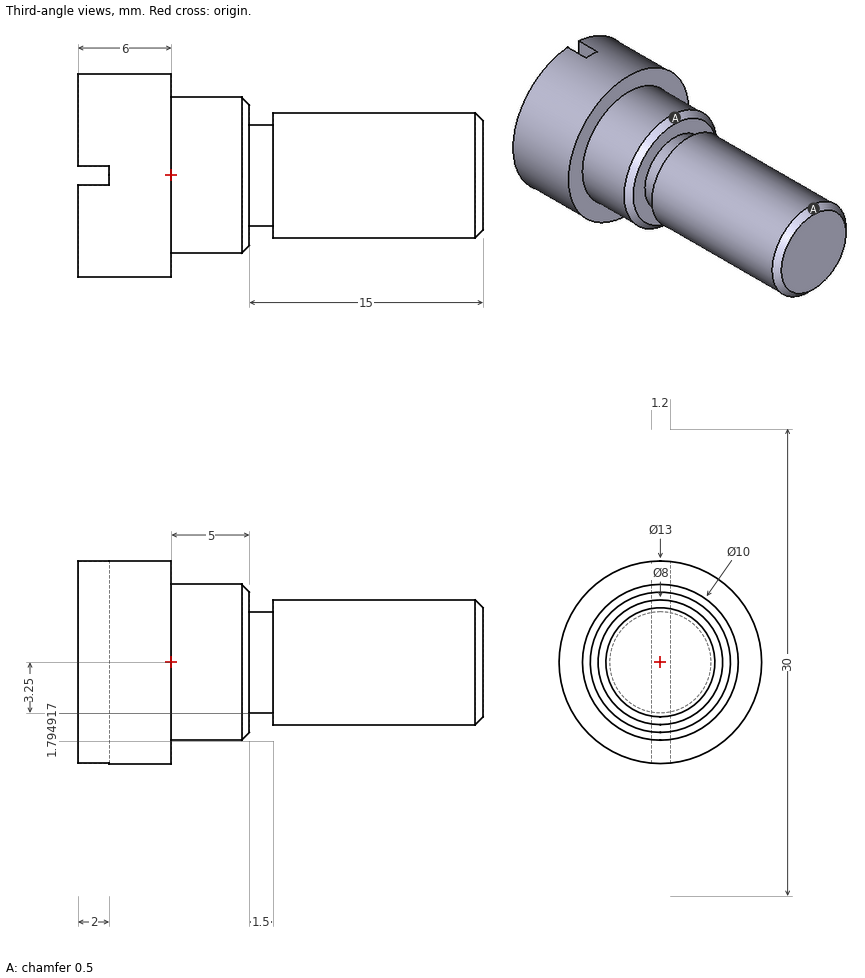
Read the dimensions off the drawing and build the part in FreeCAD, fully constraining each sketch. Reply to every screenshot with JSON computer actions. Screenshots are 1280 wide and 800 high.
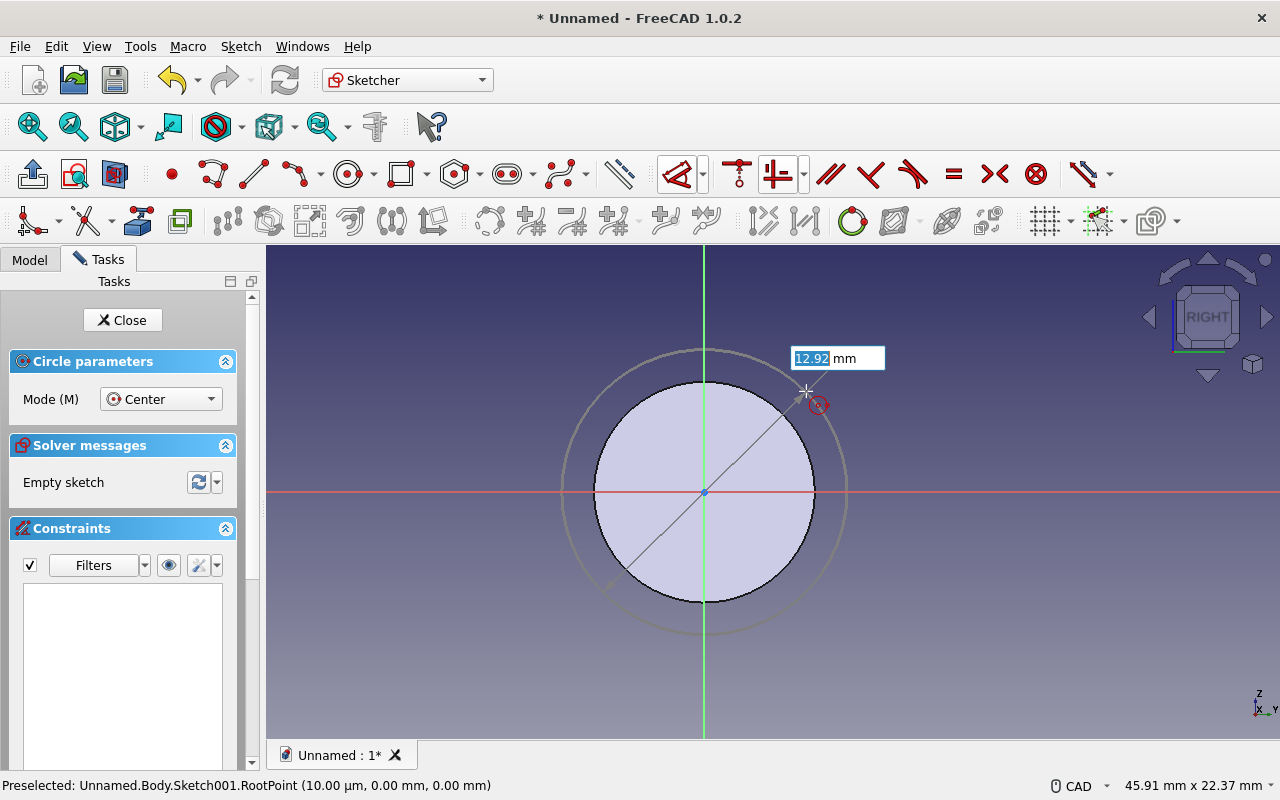
{"action": "type", "text": "13"}
{"action": "key", "text": "Return"}
{"action": "key", "text": "Escape"}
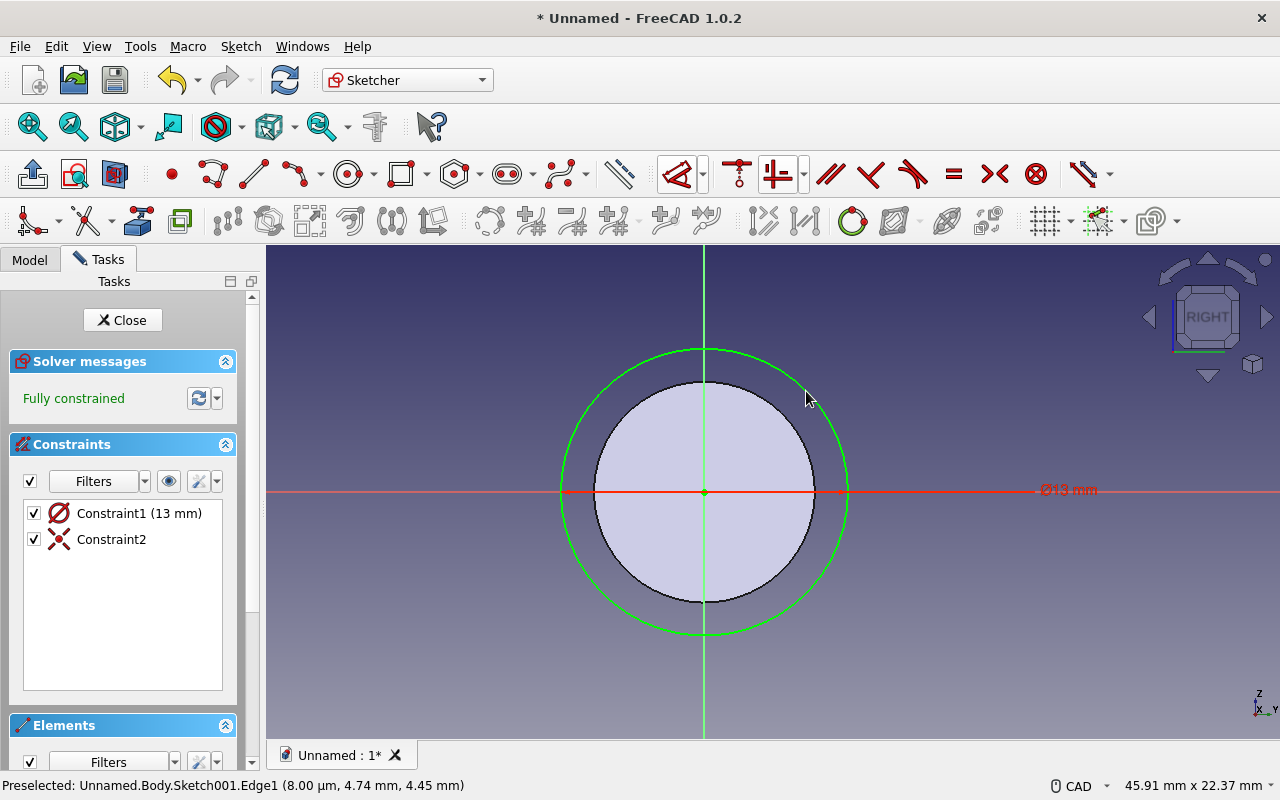
{"action": "left_click", "coordinate": [123, 320]}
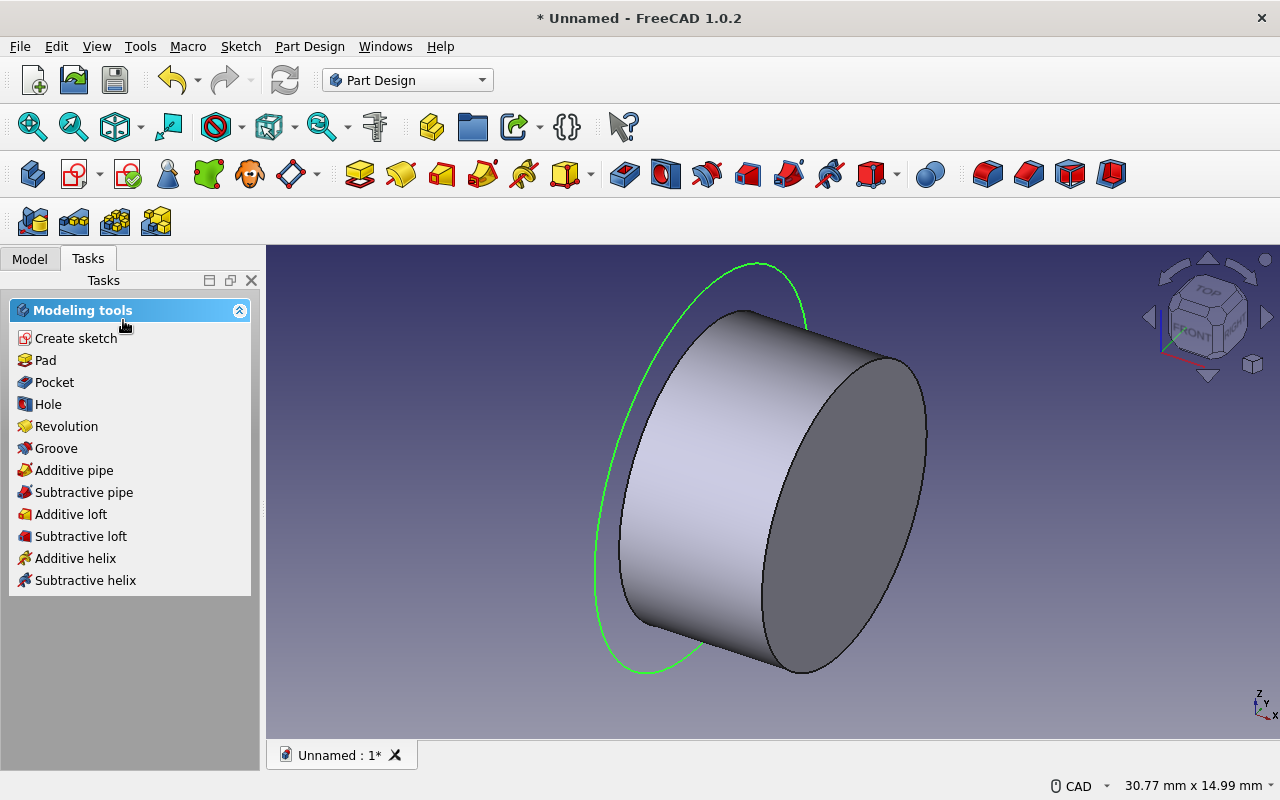
{"action": "left_click", "coordinate": [360, 174]}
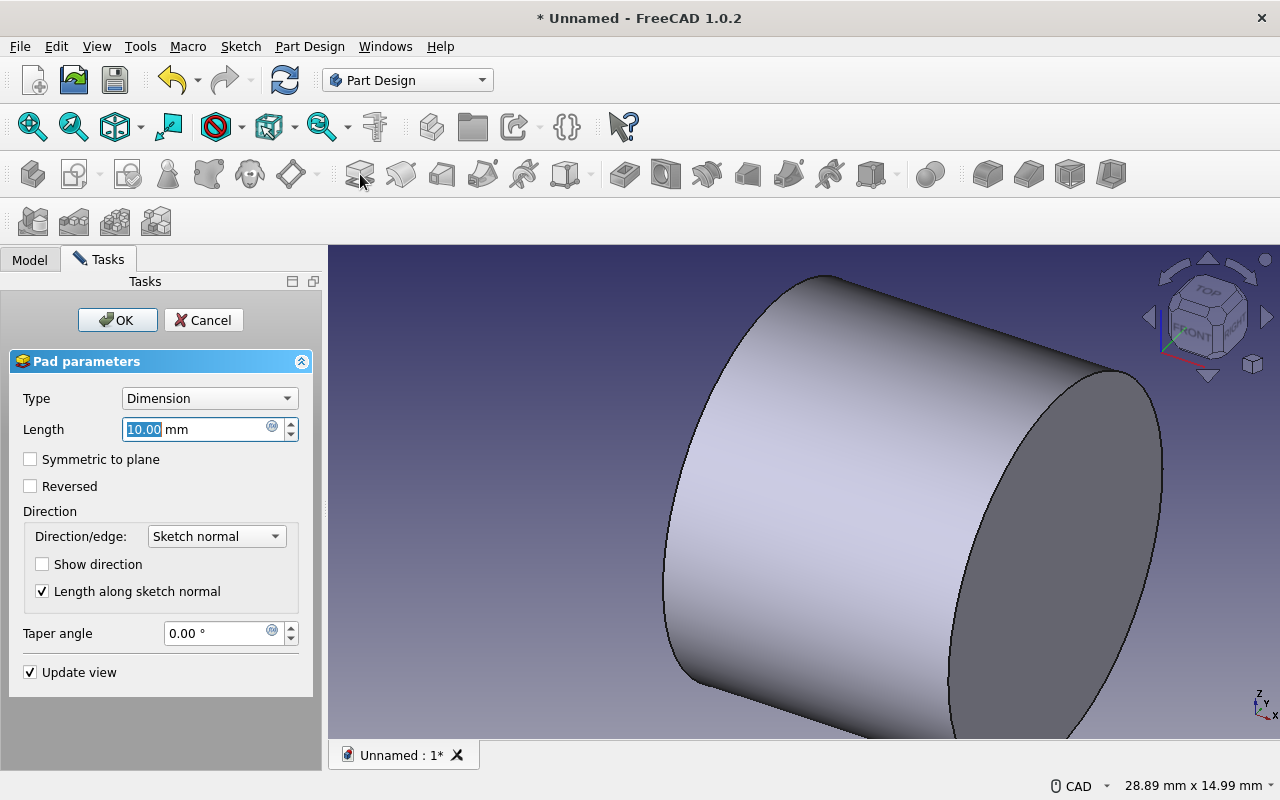
{"action": "type", "text": "6"}
{"action": "key", "text": "Tab"}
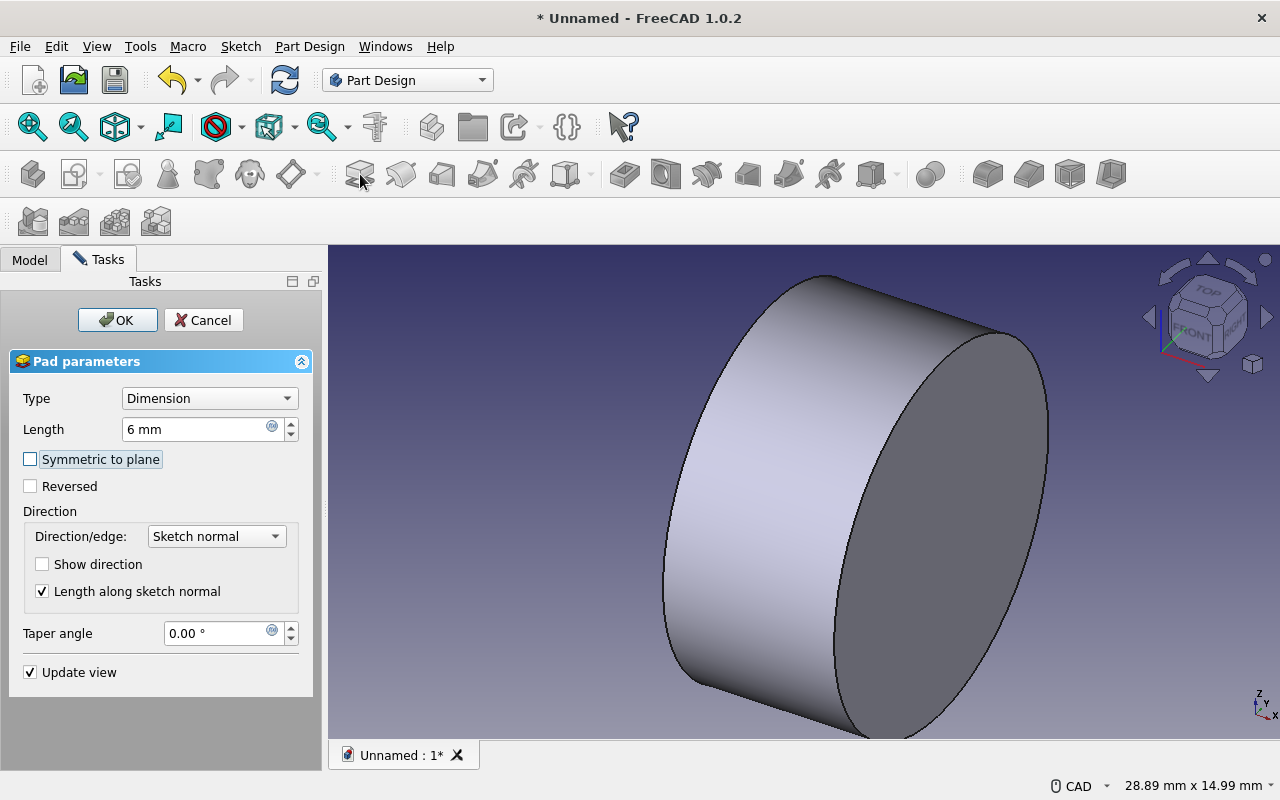
{"action": "left_click", "coordinate": [31, 486]}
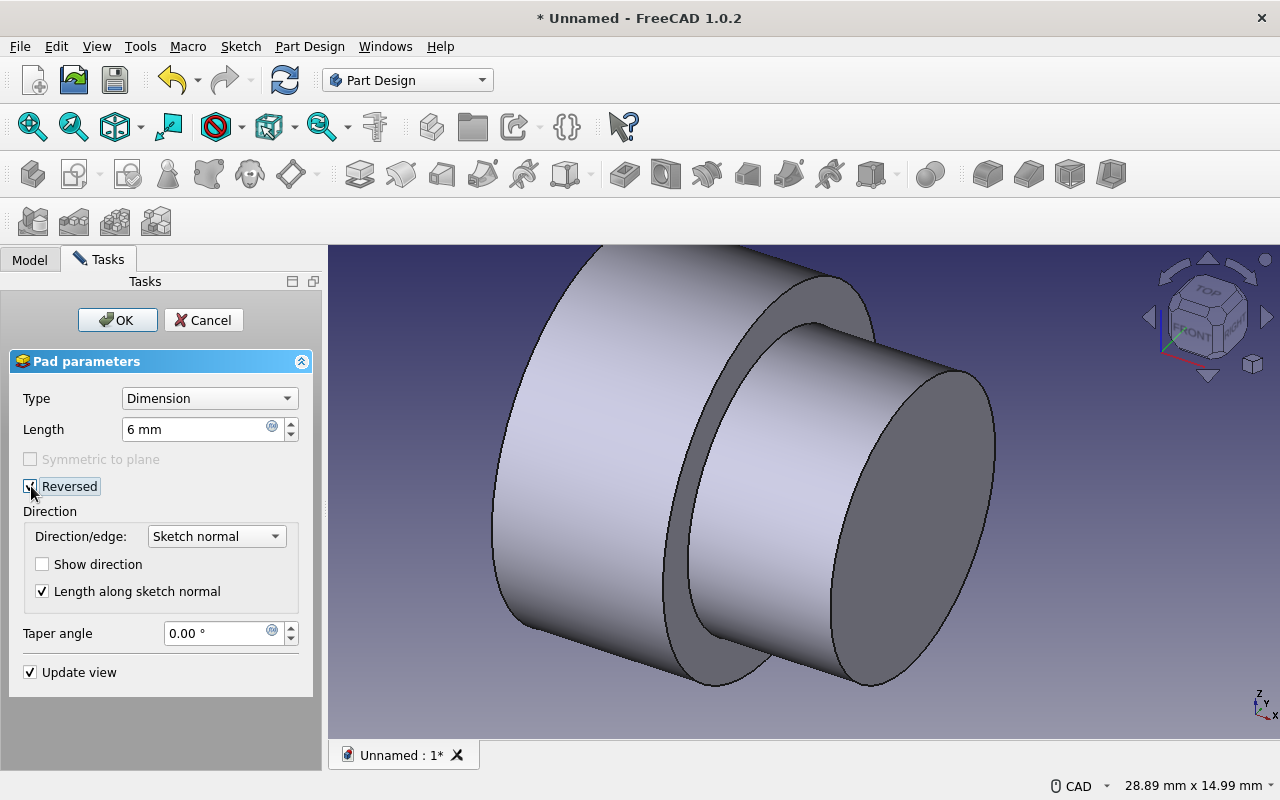
{"action": "left_click", "coordinate": [118, 320]}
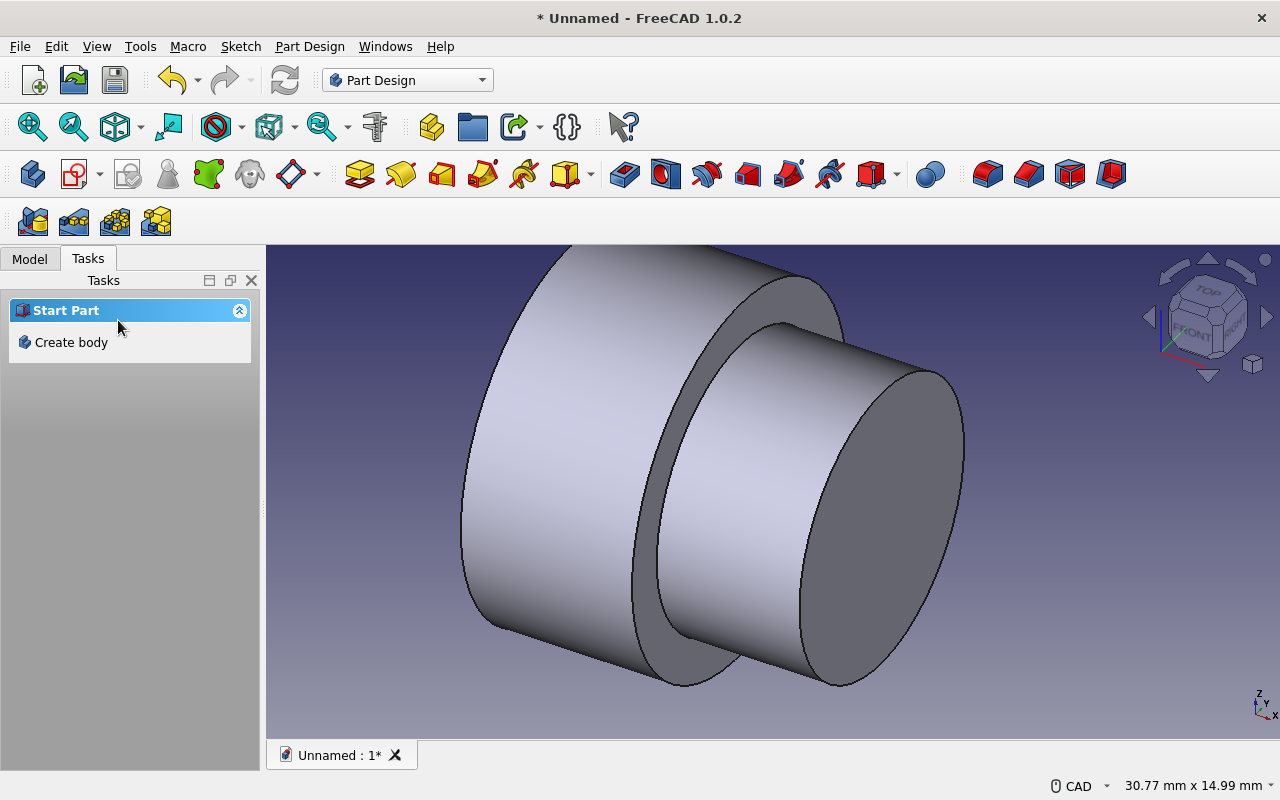
{"action": "left_click", "coordinate": [33, 128]}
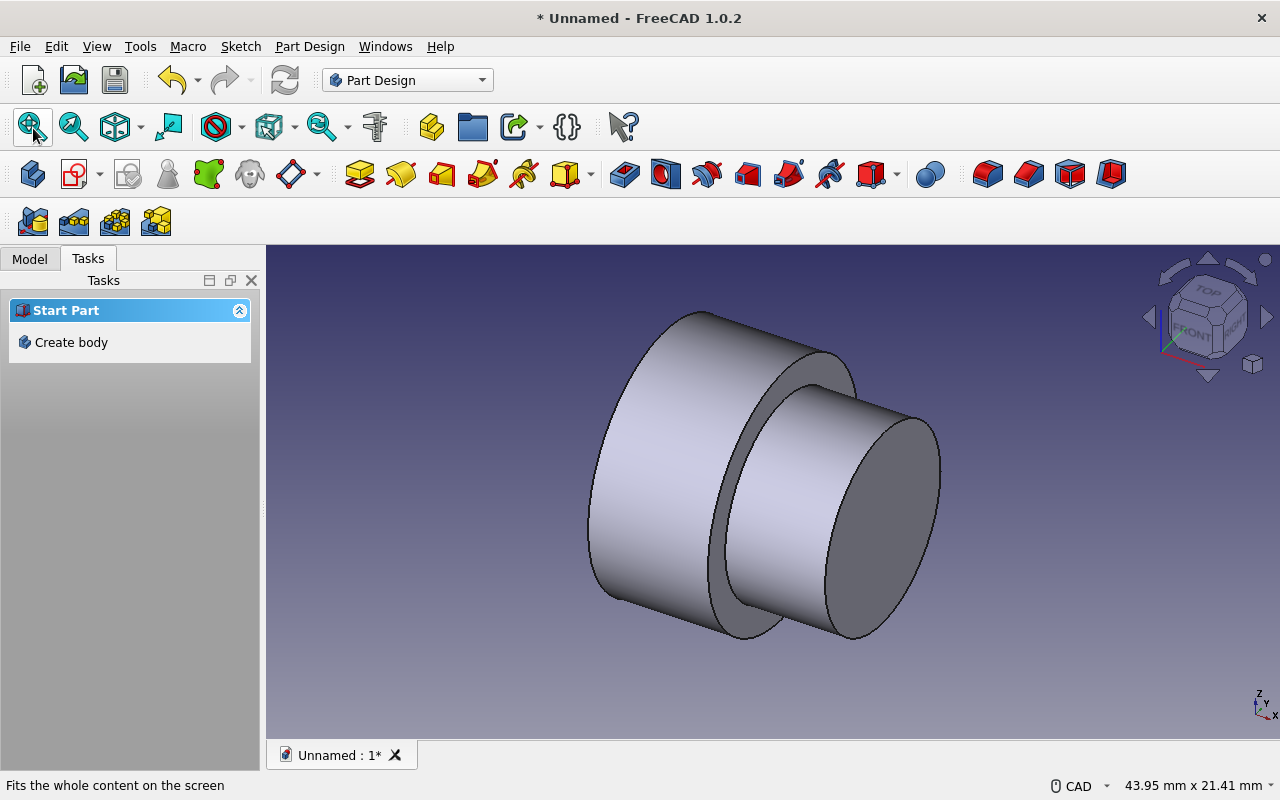
{"action": "key", "text": "6"}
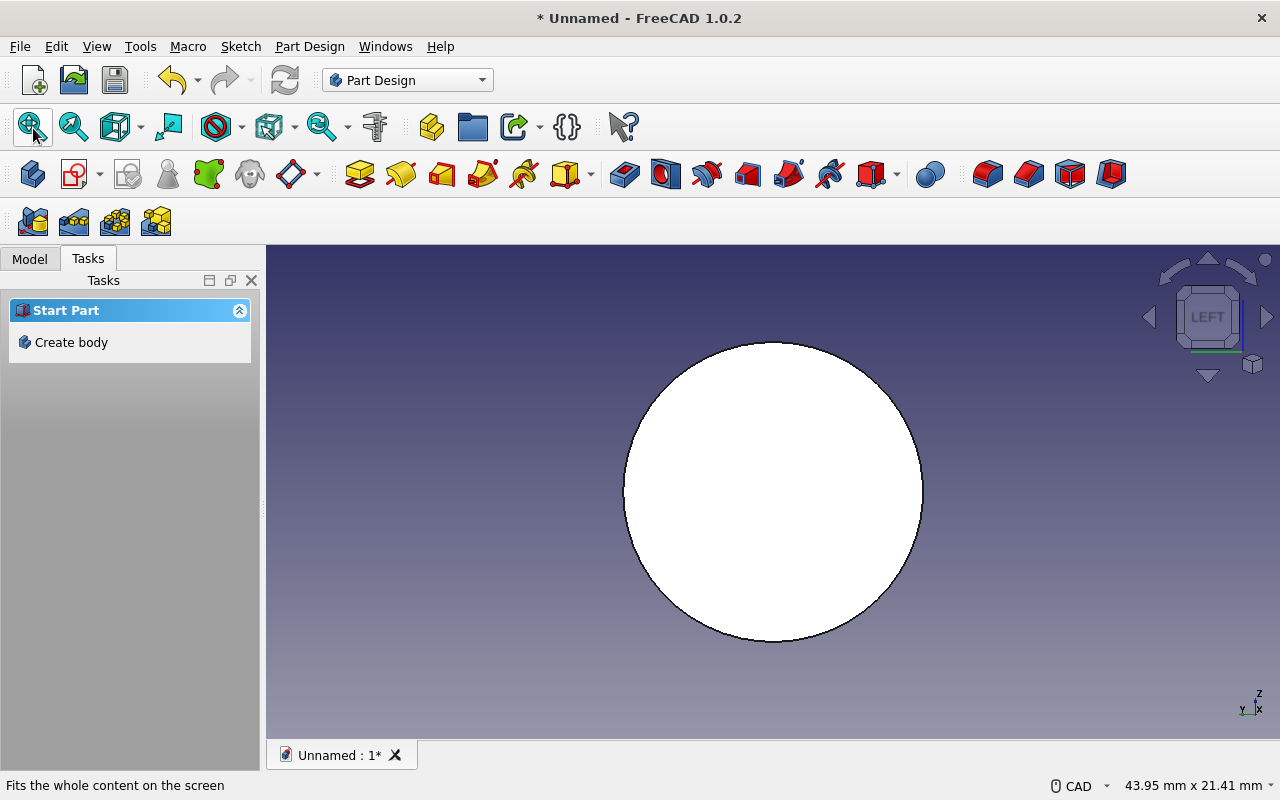
{"action": "left_click", "coordinate": [773, 491]}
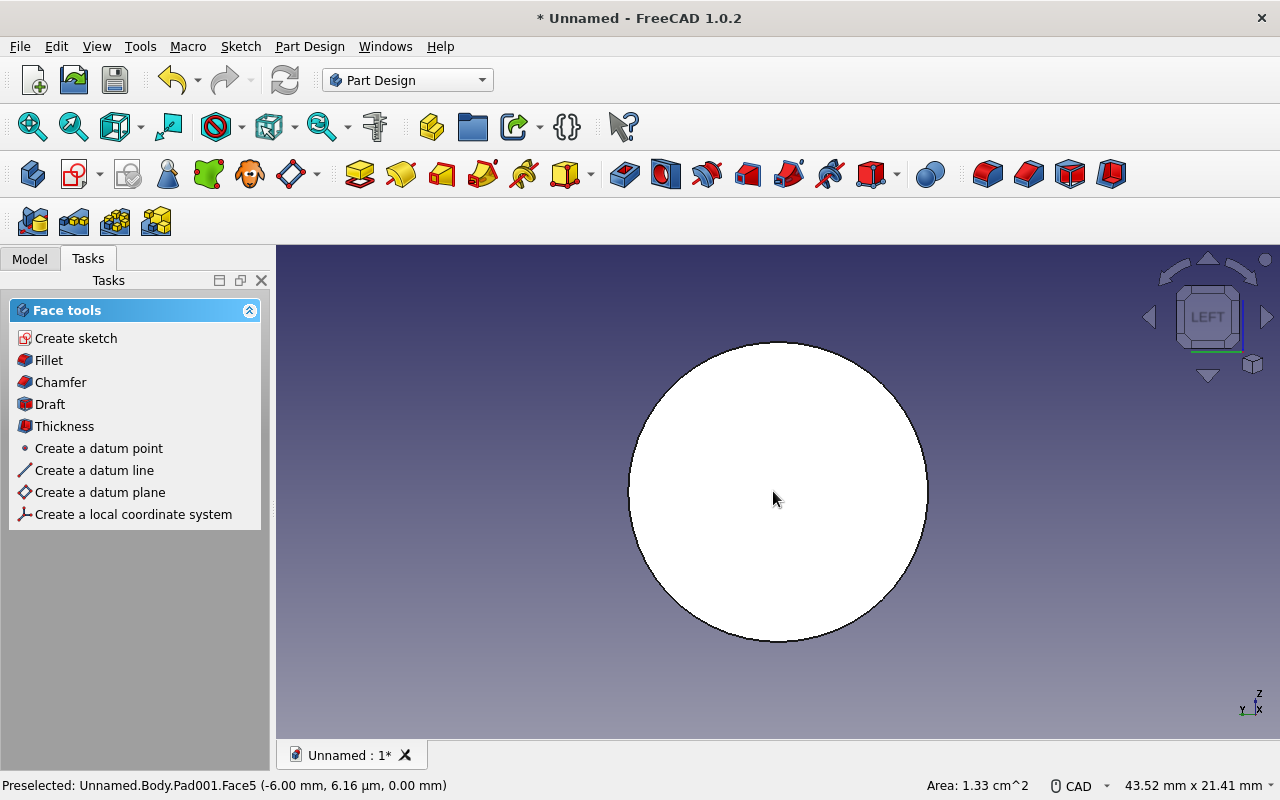
{"action": "left_click", "coordinate": [74, 174]}